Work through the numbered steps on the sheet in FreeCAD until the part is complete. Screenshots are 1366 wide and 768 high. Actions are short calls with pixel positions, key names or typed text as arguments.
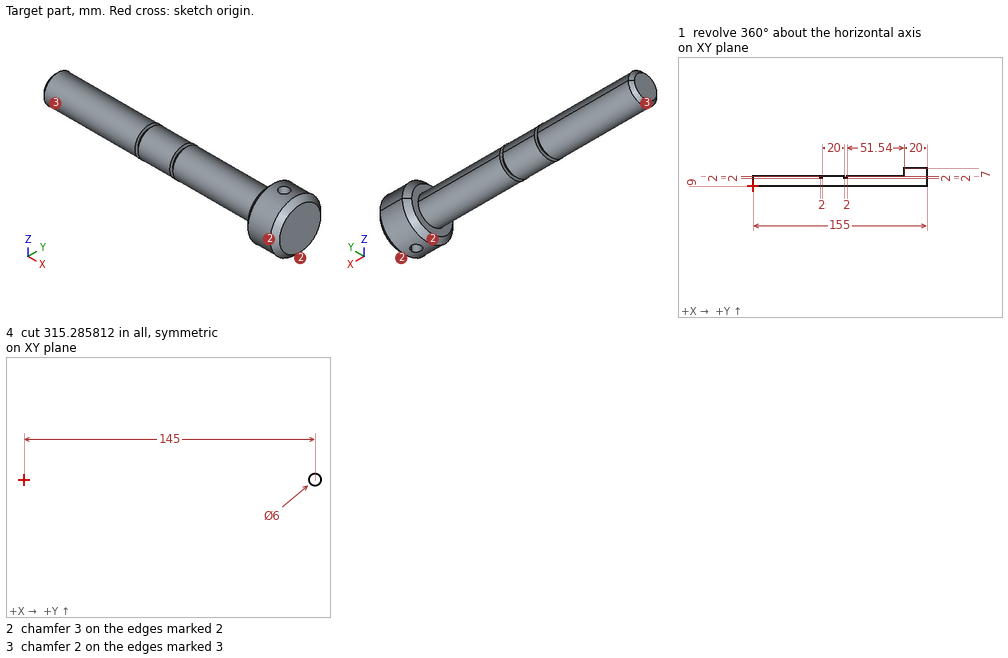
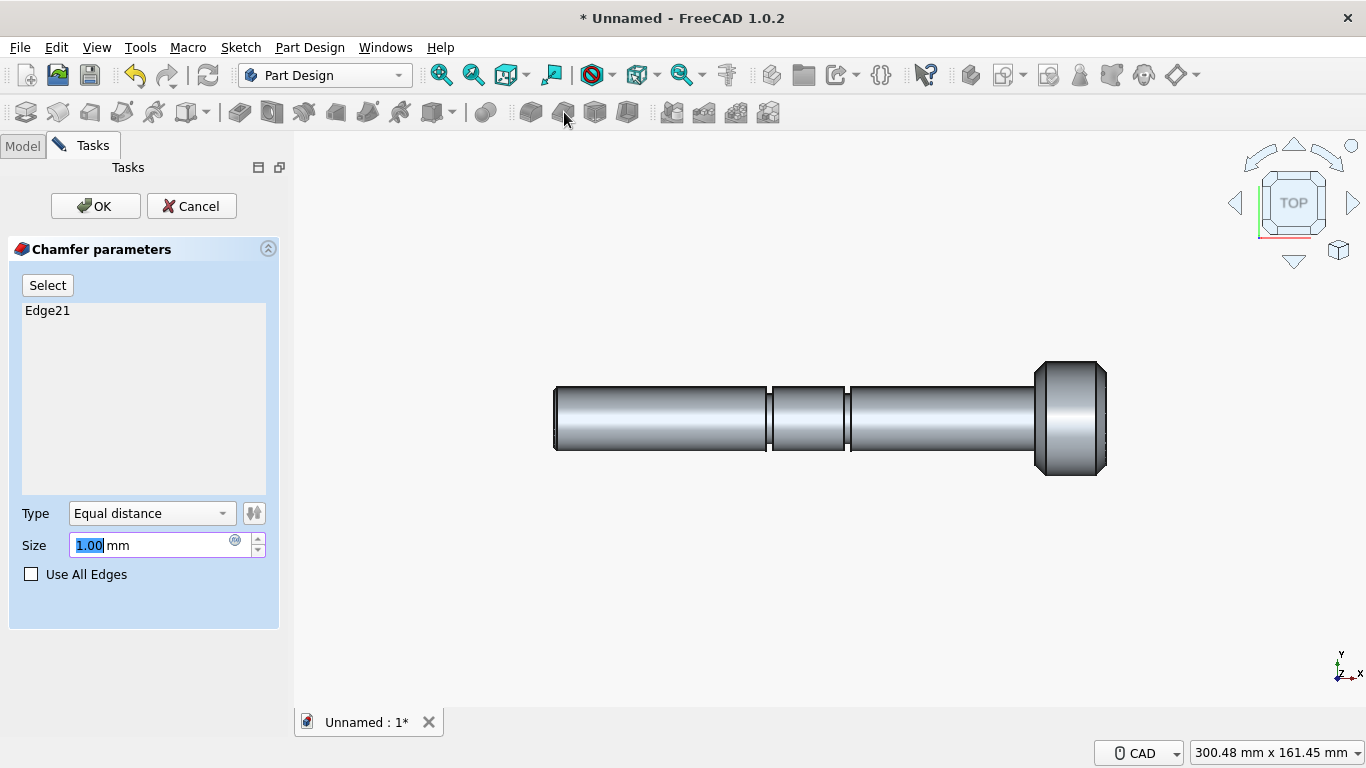
text(2)
key(Tab)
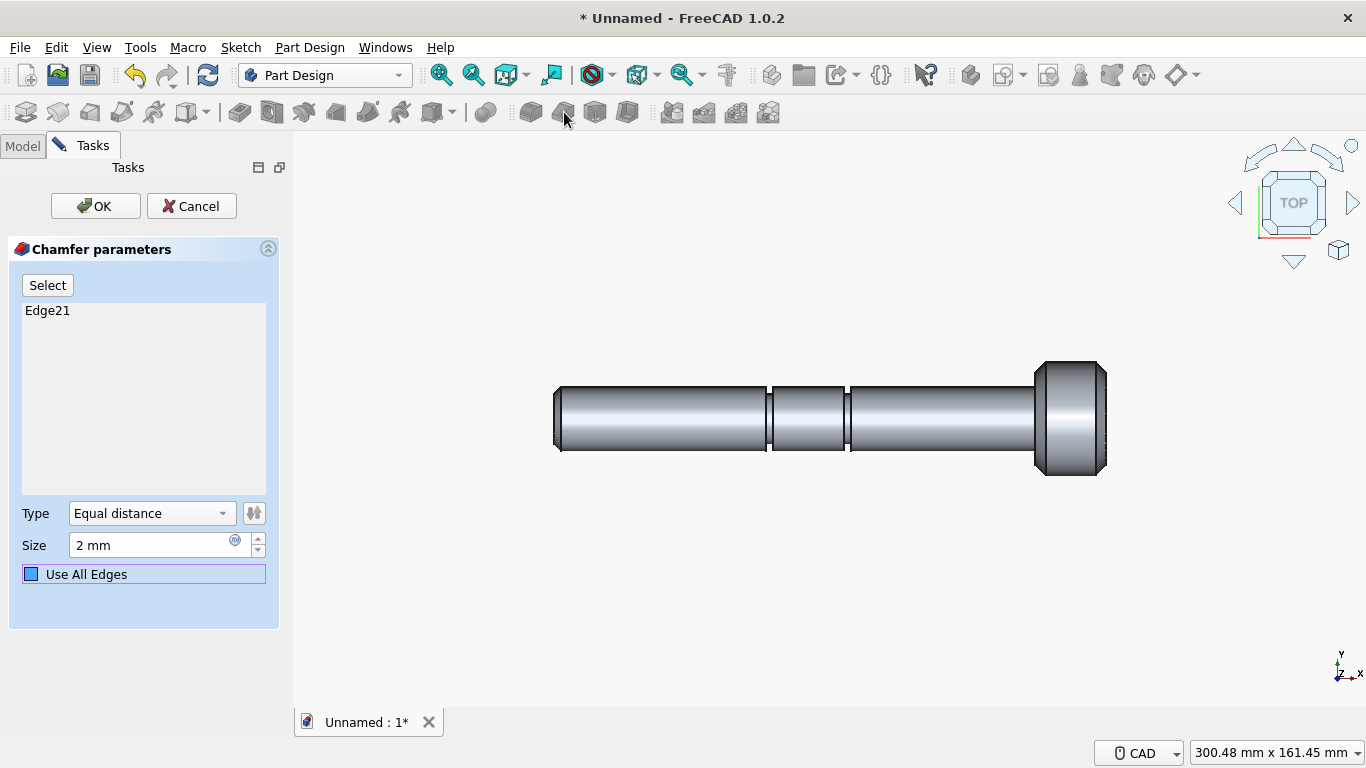
click(96, 206)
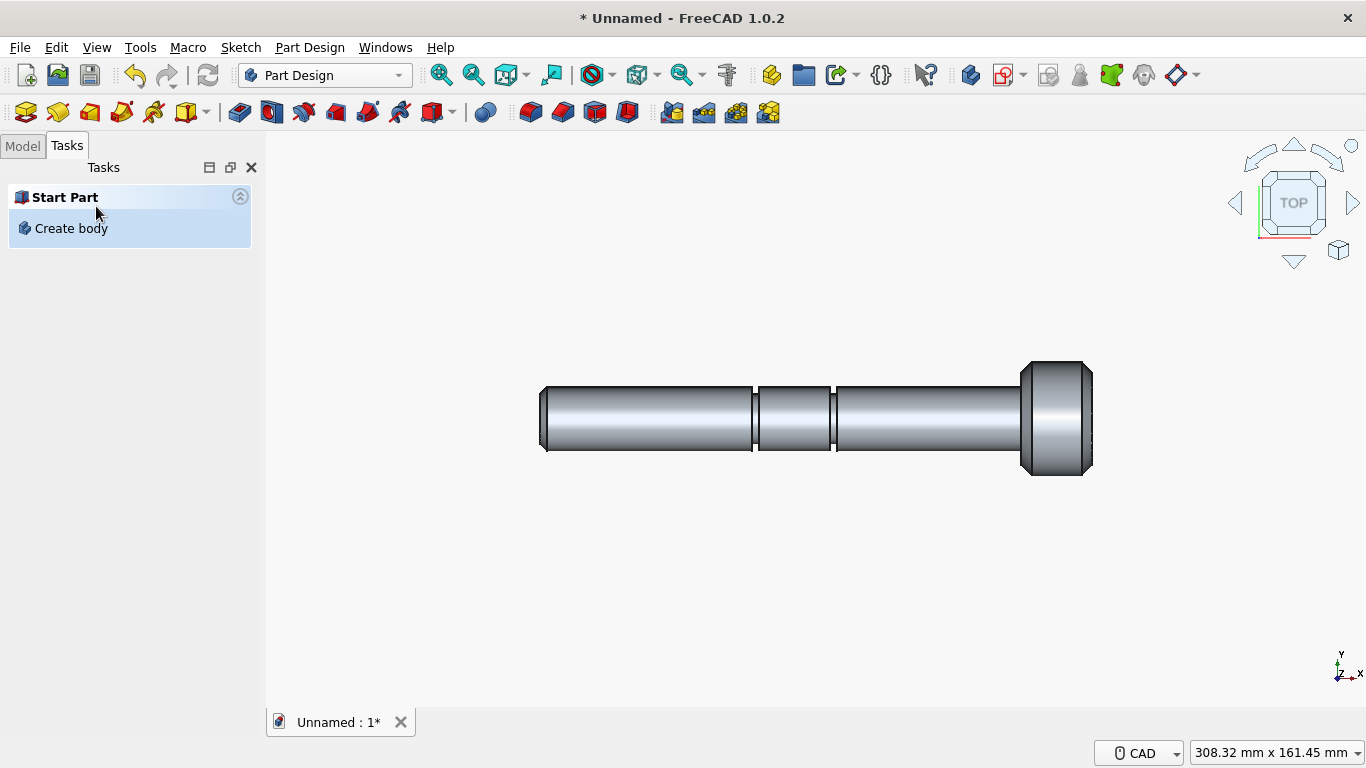
click(1004, 76)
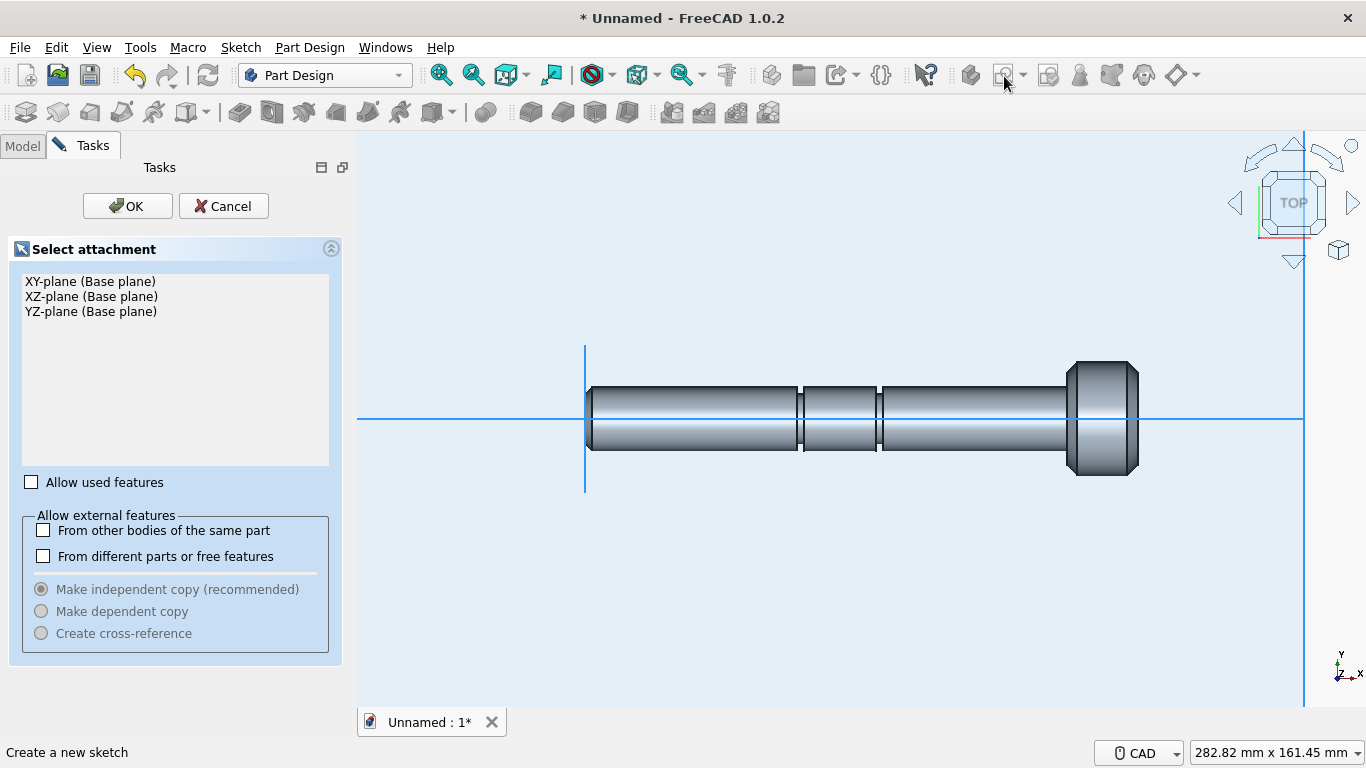
click(82, 282)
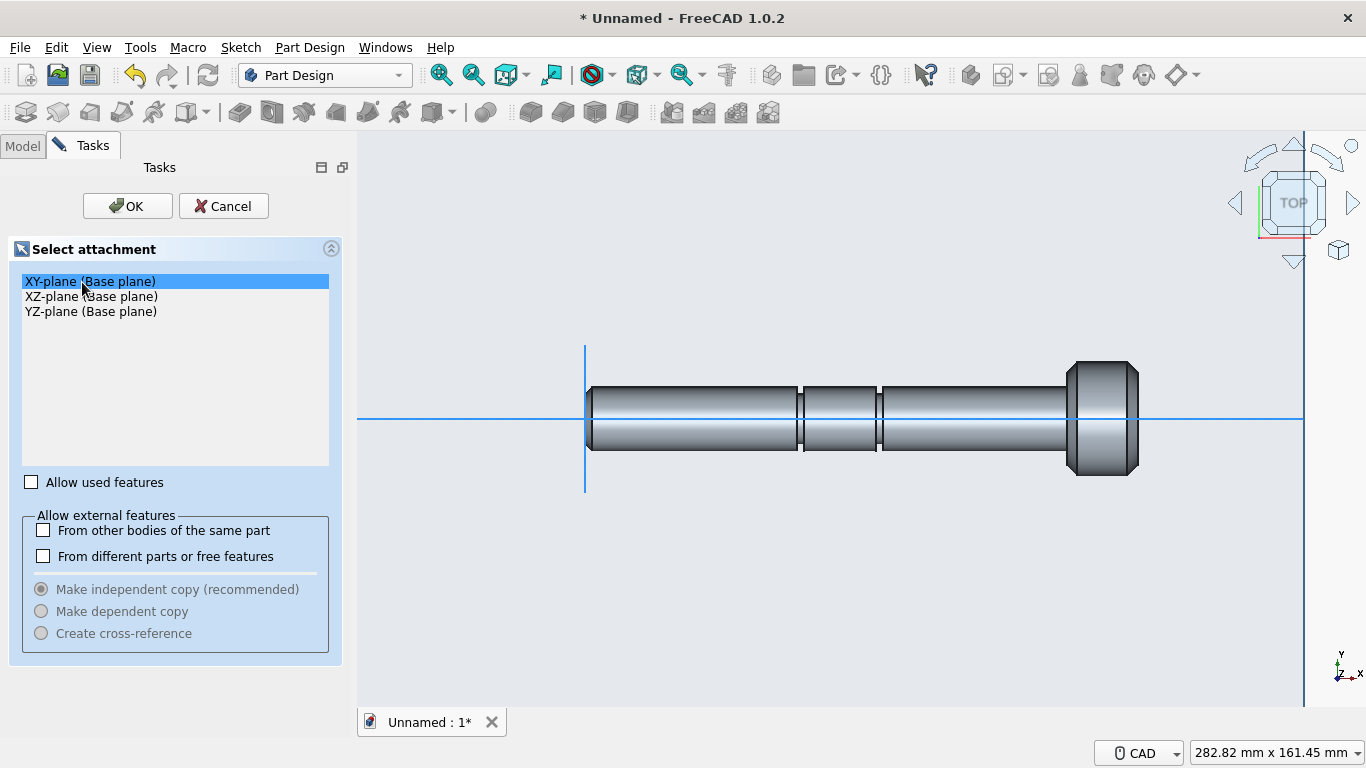
click(128, 206)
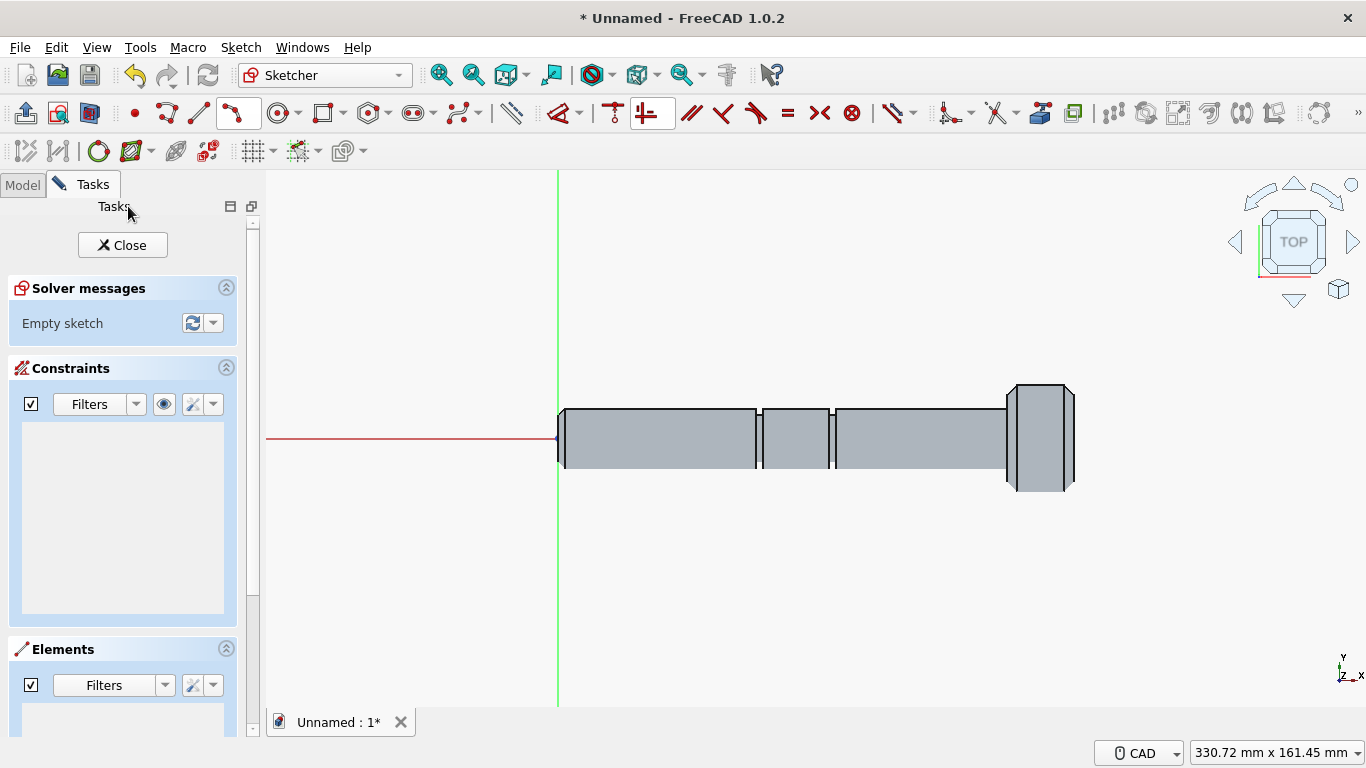
click(90, 114)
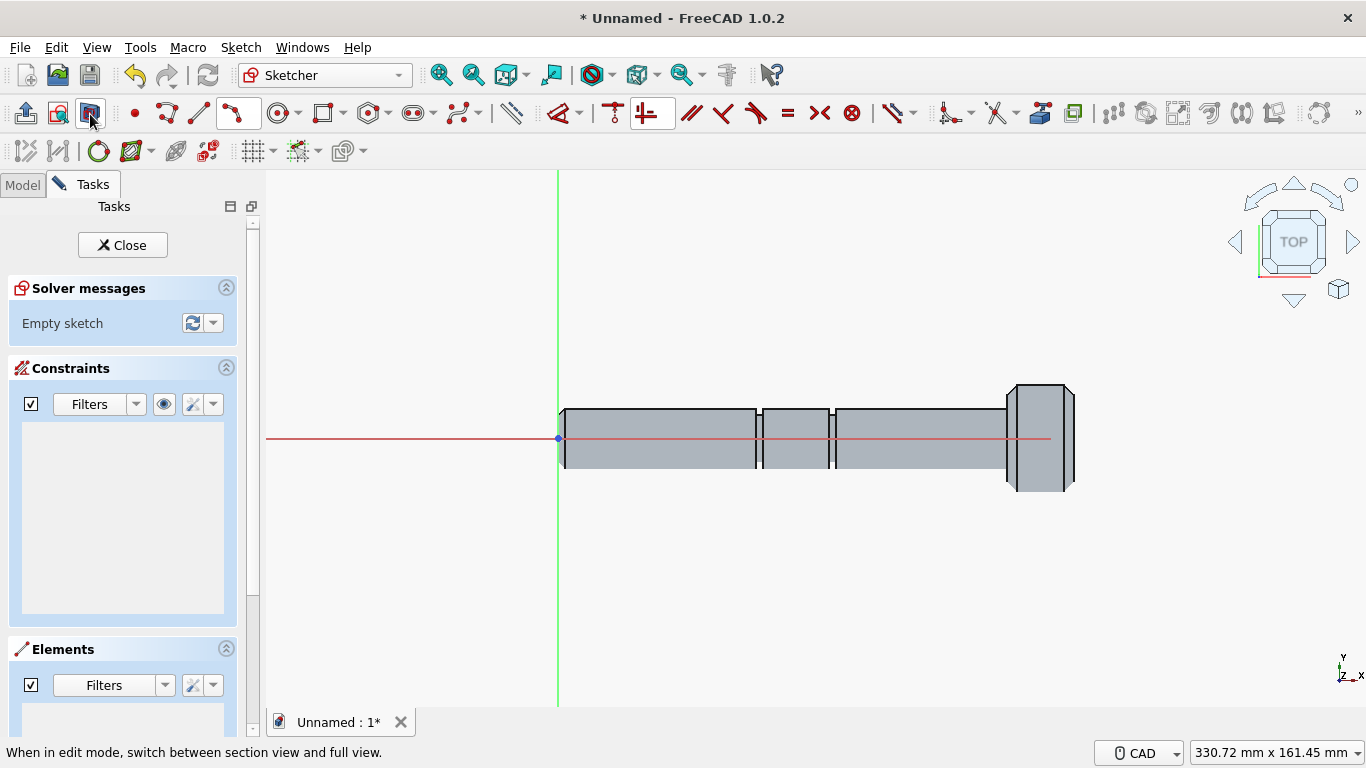
scroll(1059, 439, up, 14)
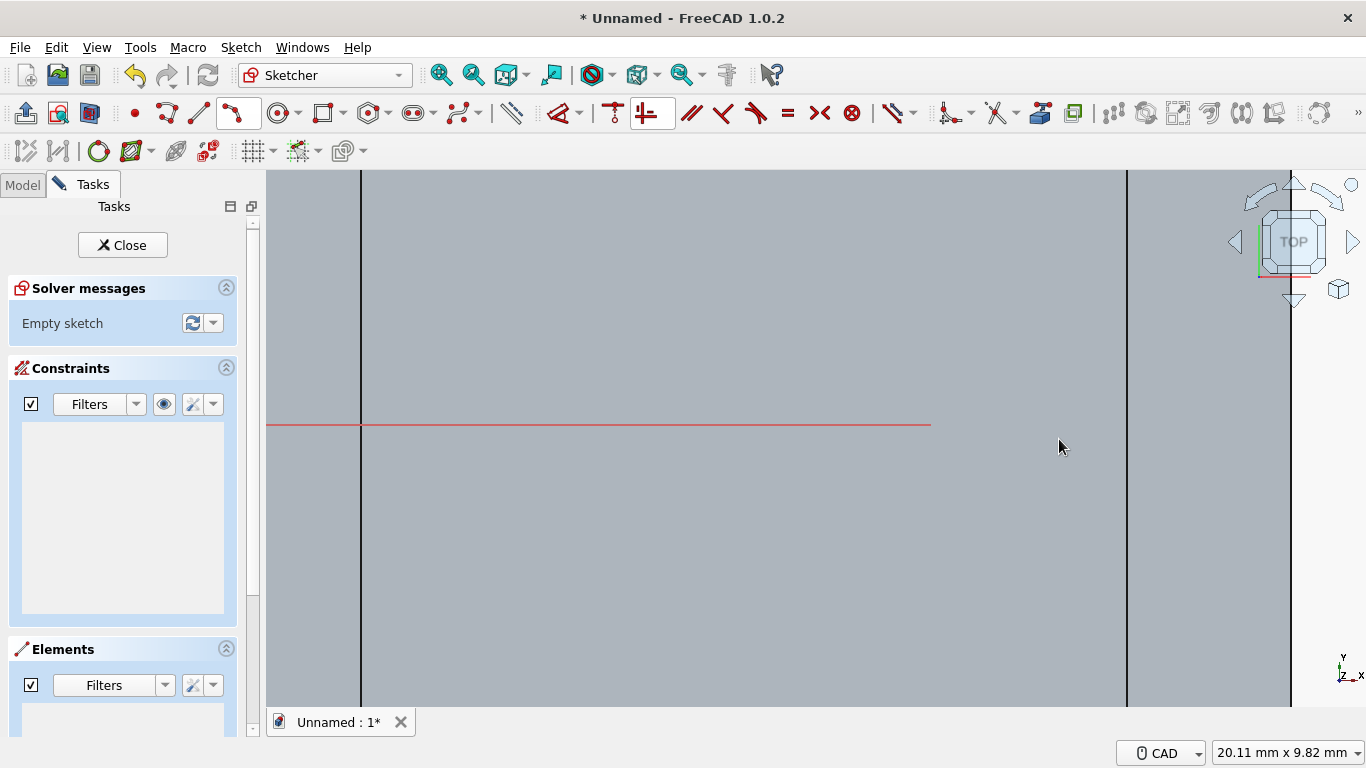
click(278, 114)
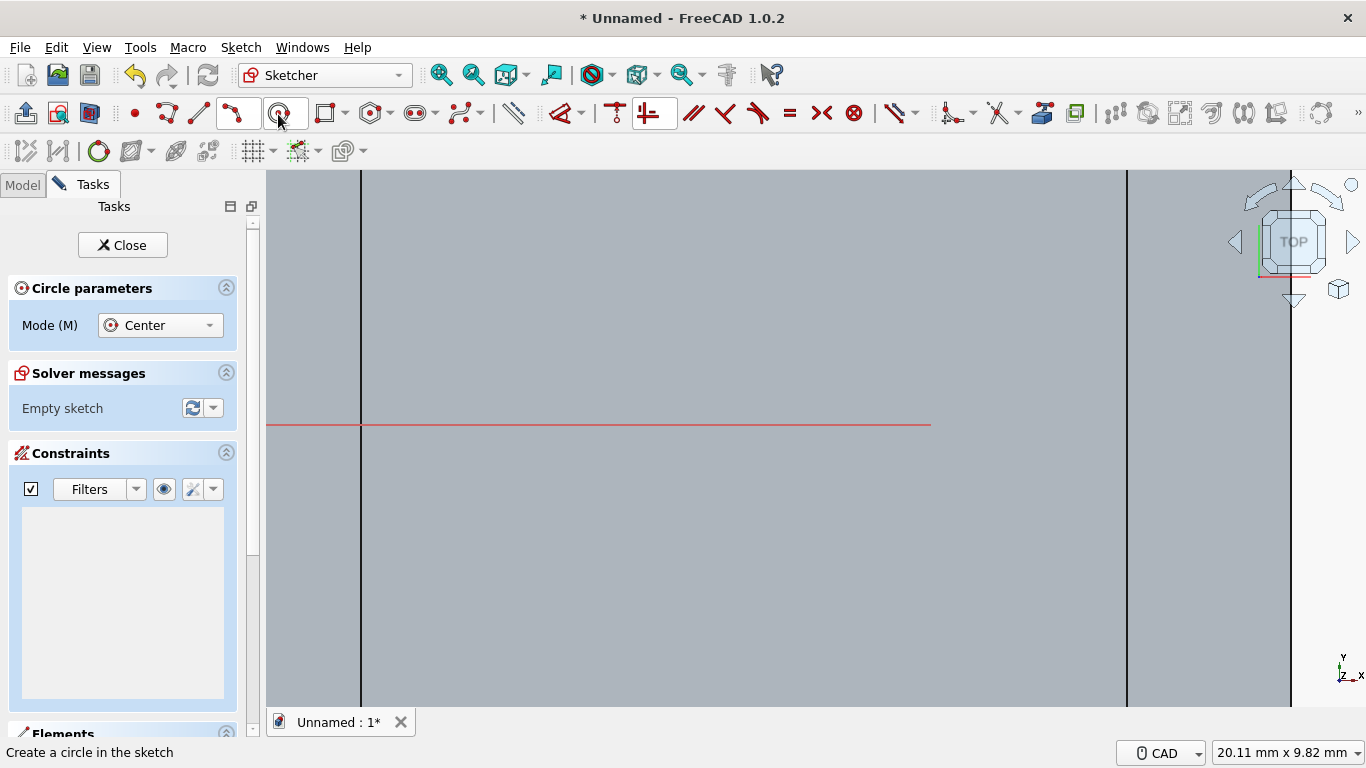
click(744, 425)
move(860, 309)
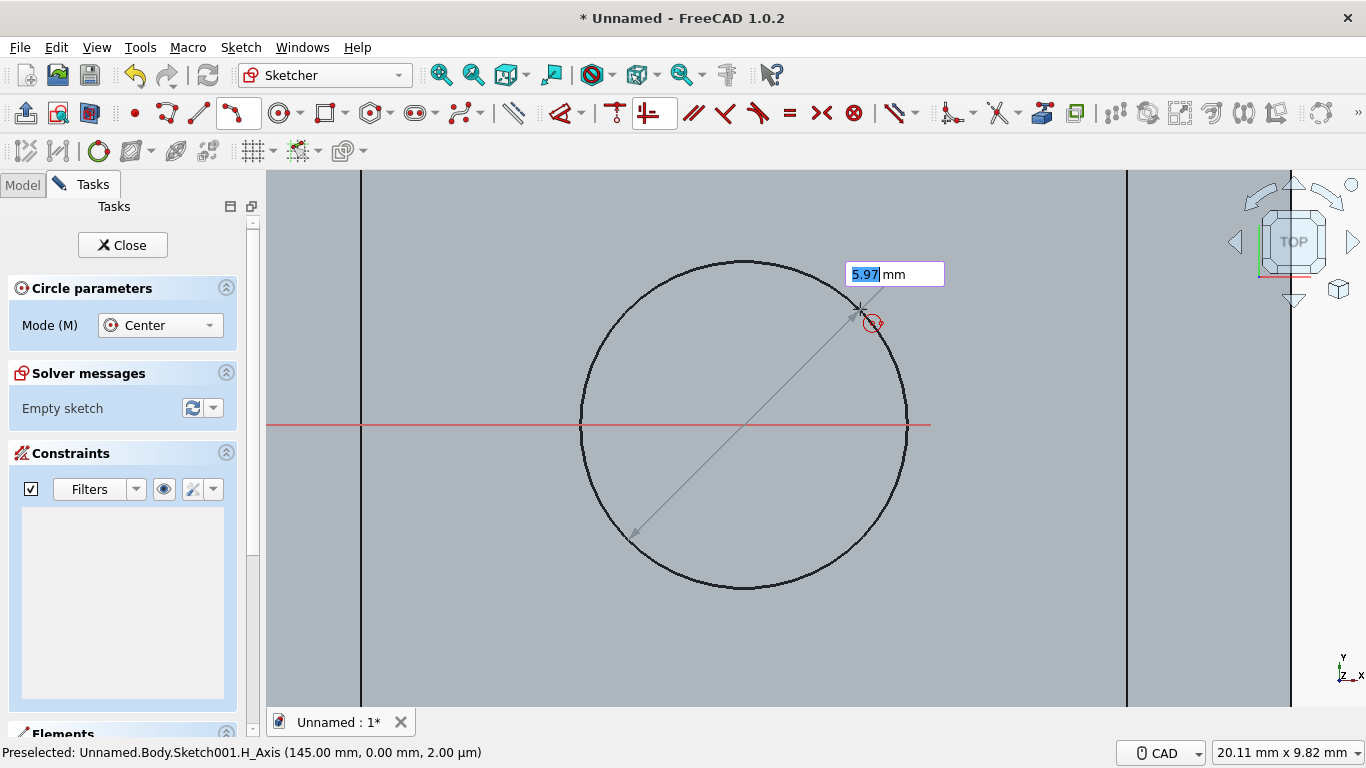
text(6)
key(Return)
key(Escape)